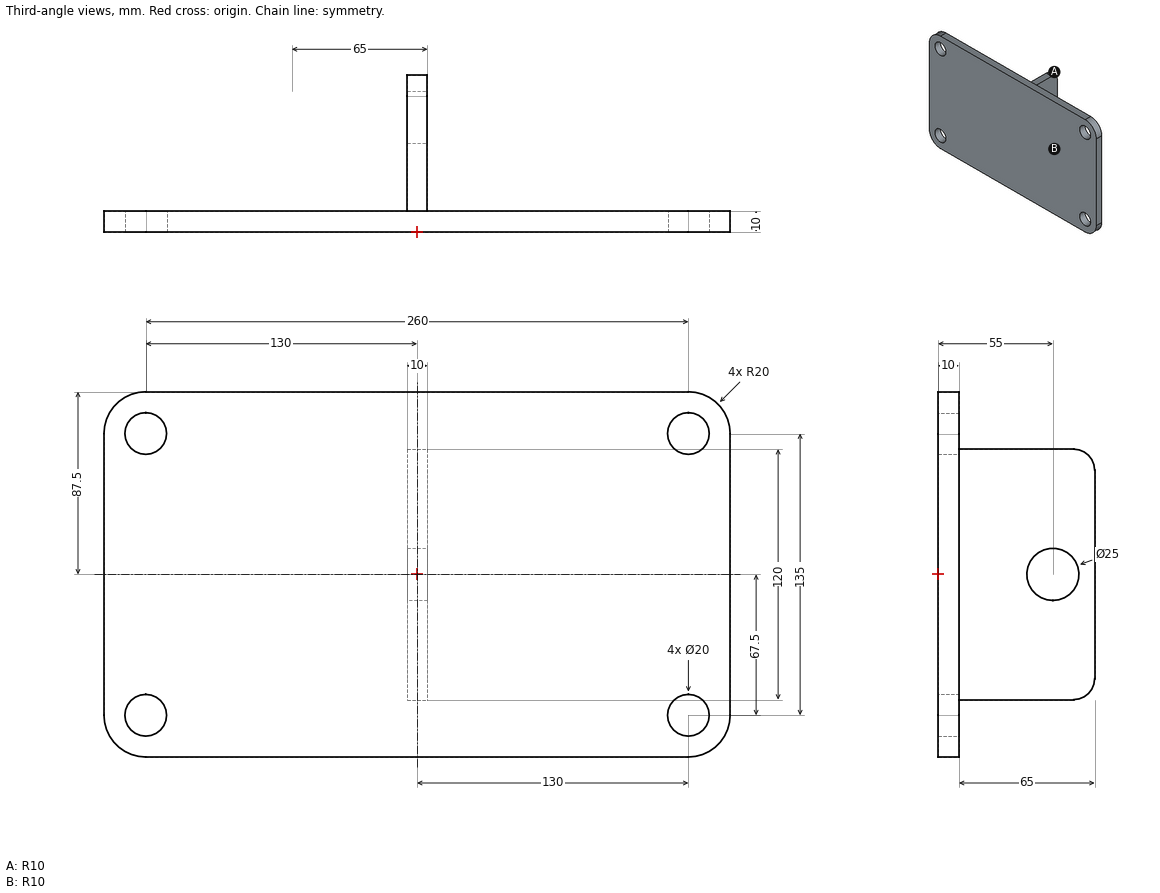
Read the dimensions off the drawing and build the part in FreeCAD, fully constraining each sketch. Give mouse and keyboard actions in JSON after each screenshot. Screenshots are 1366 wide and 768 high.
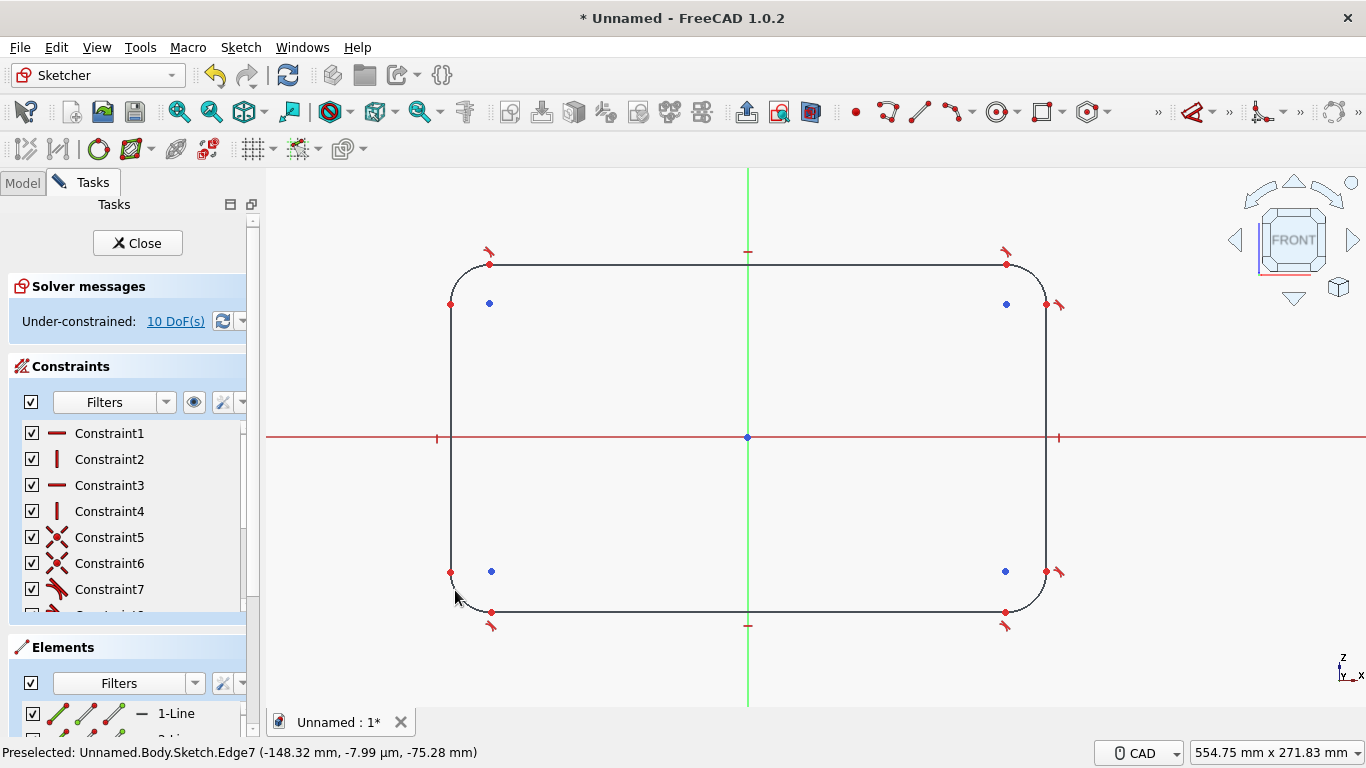
{"action": "left_click", "coordinate": [451, 492]}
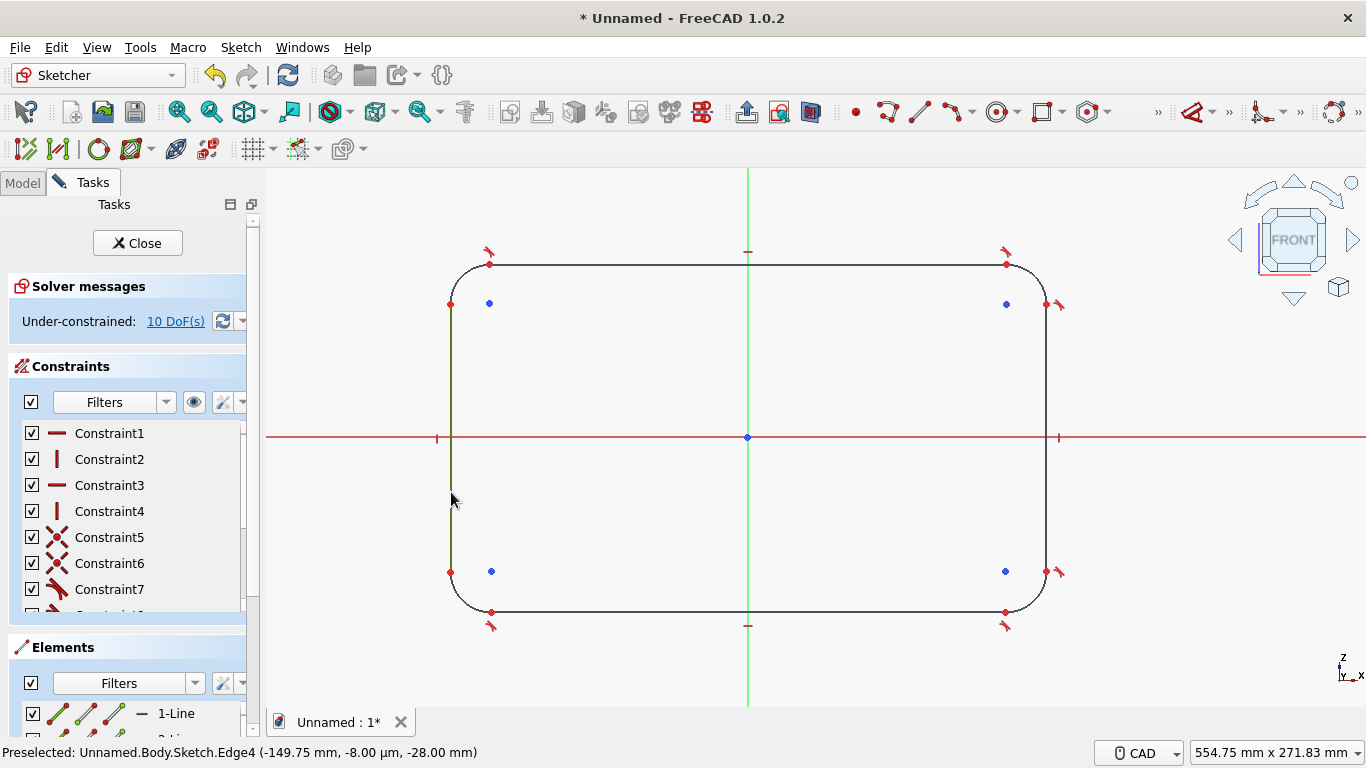
{"action": "left_click", "coordinate": [455, 591]}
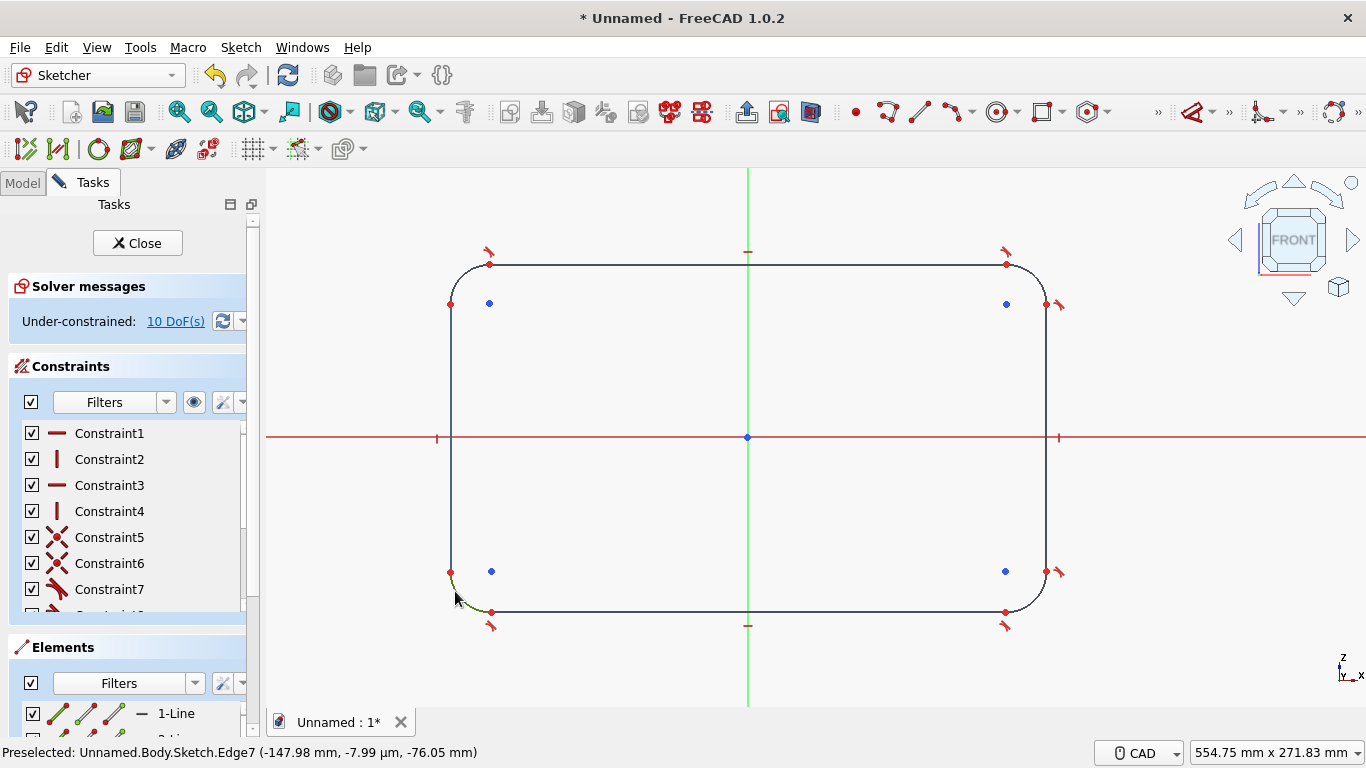
{"action": "key", "text": "t"}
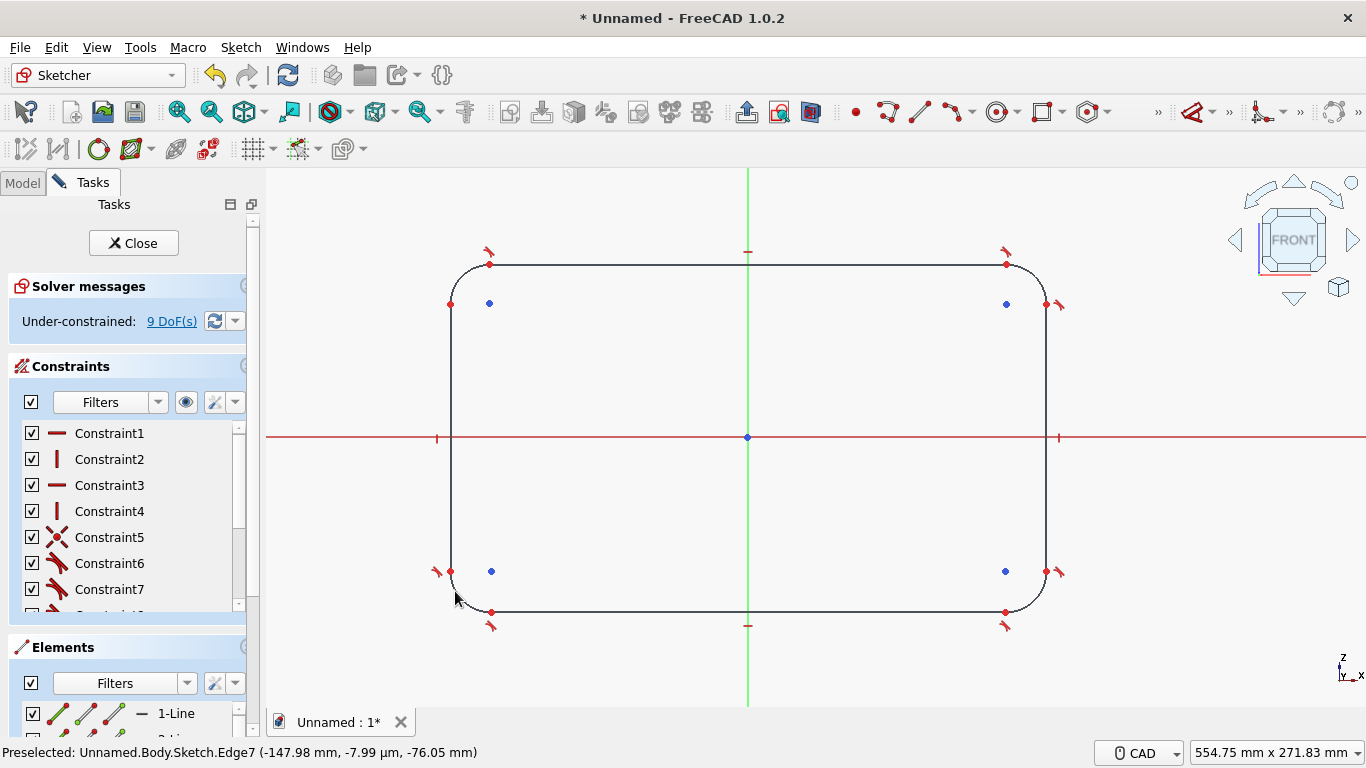
{"action": "left_click", "coordinate": [451, 491]}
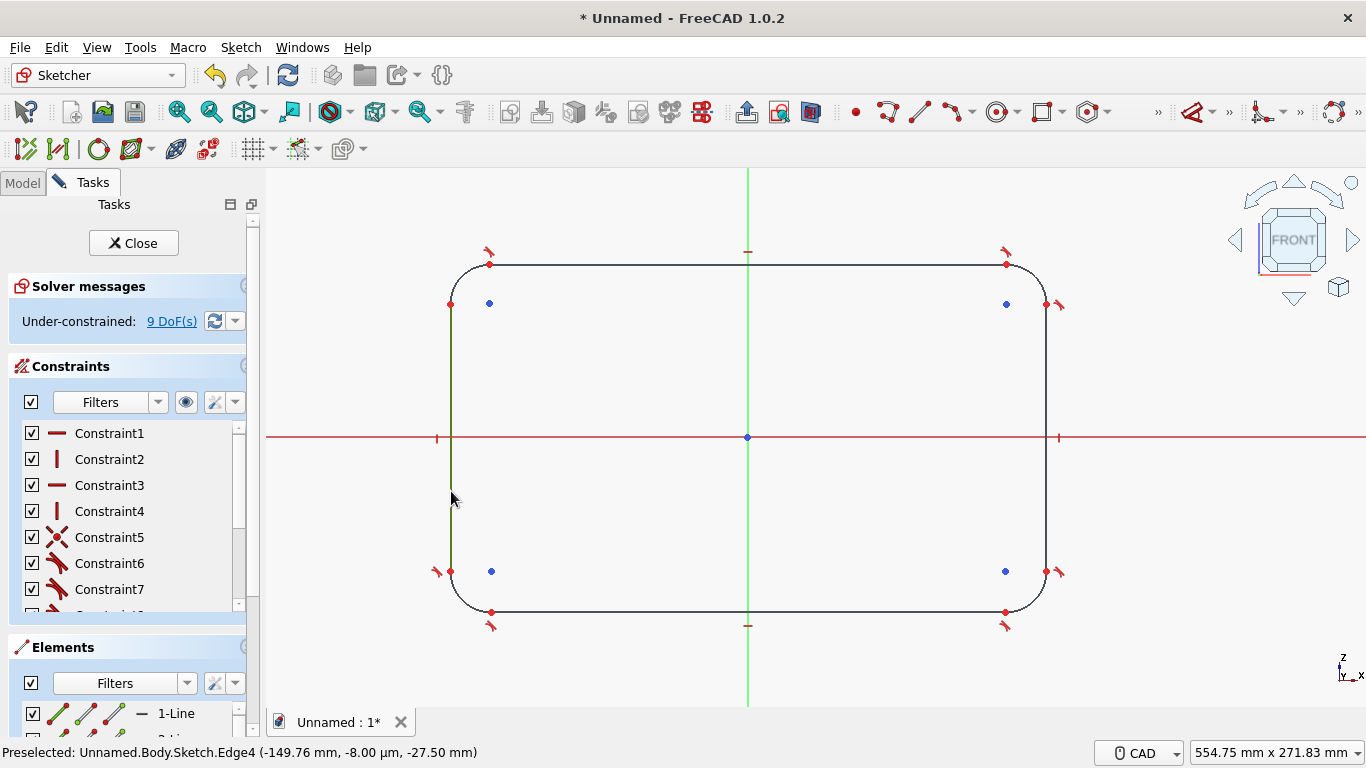
{"action": "left_click", "coordinate": [472, 269]}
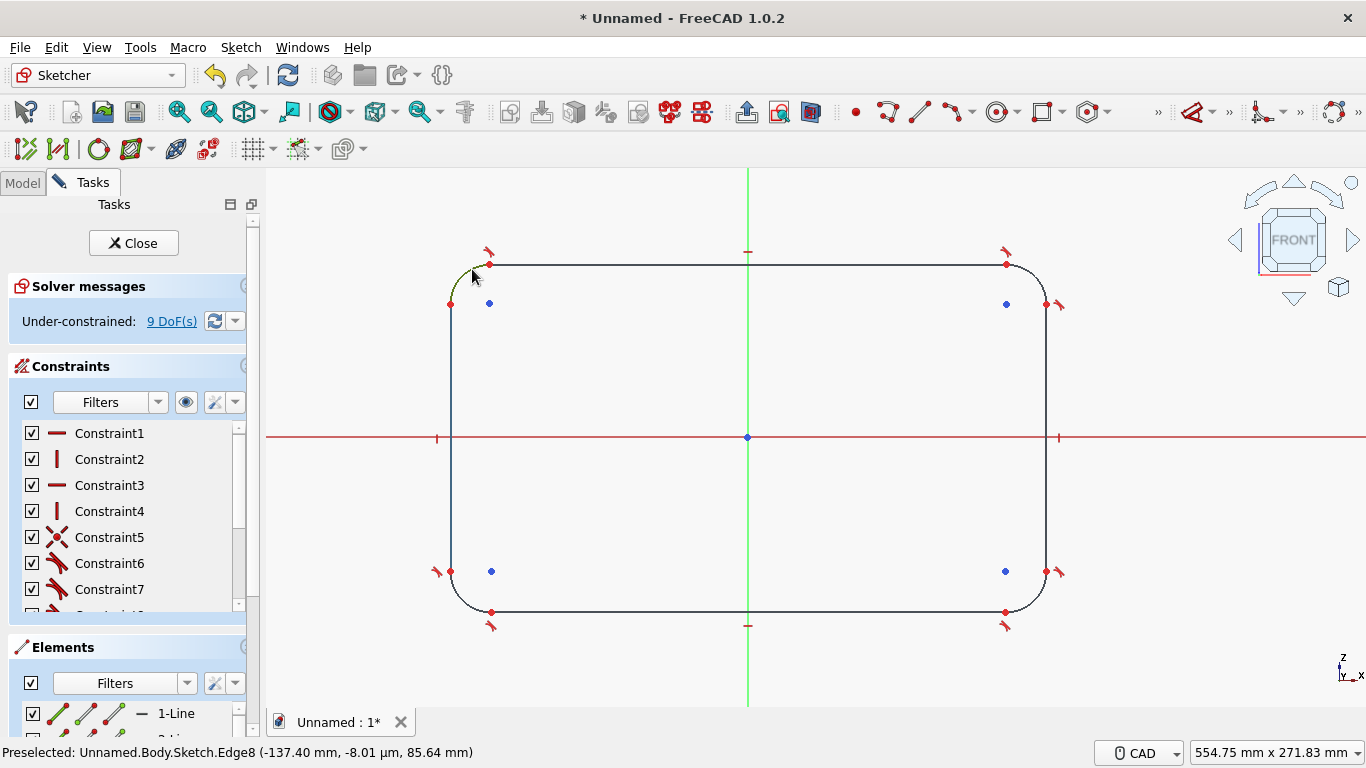
{"action": "key", "text": "t"}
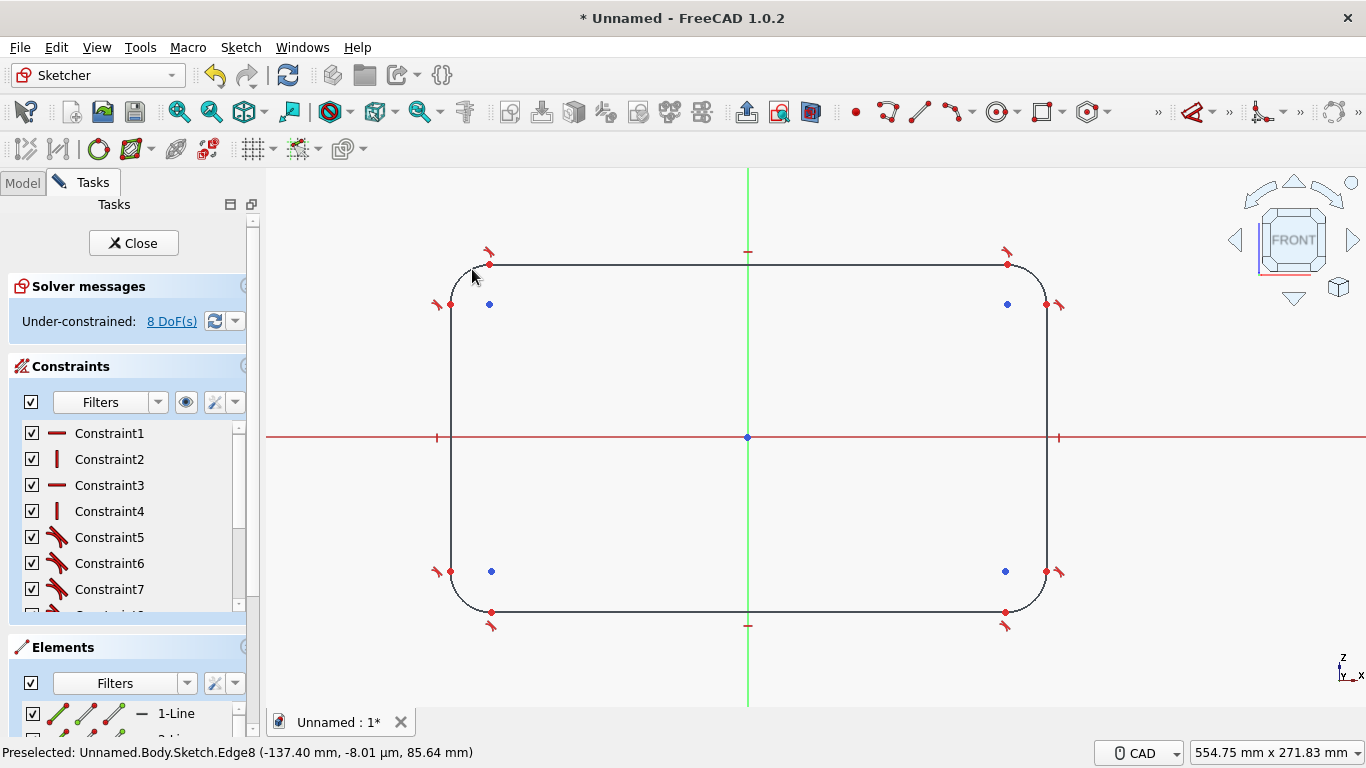
{"action": "left_click", "coordinate": [1042, 286]}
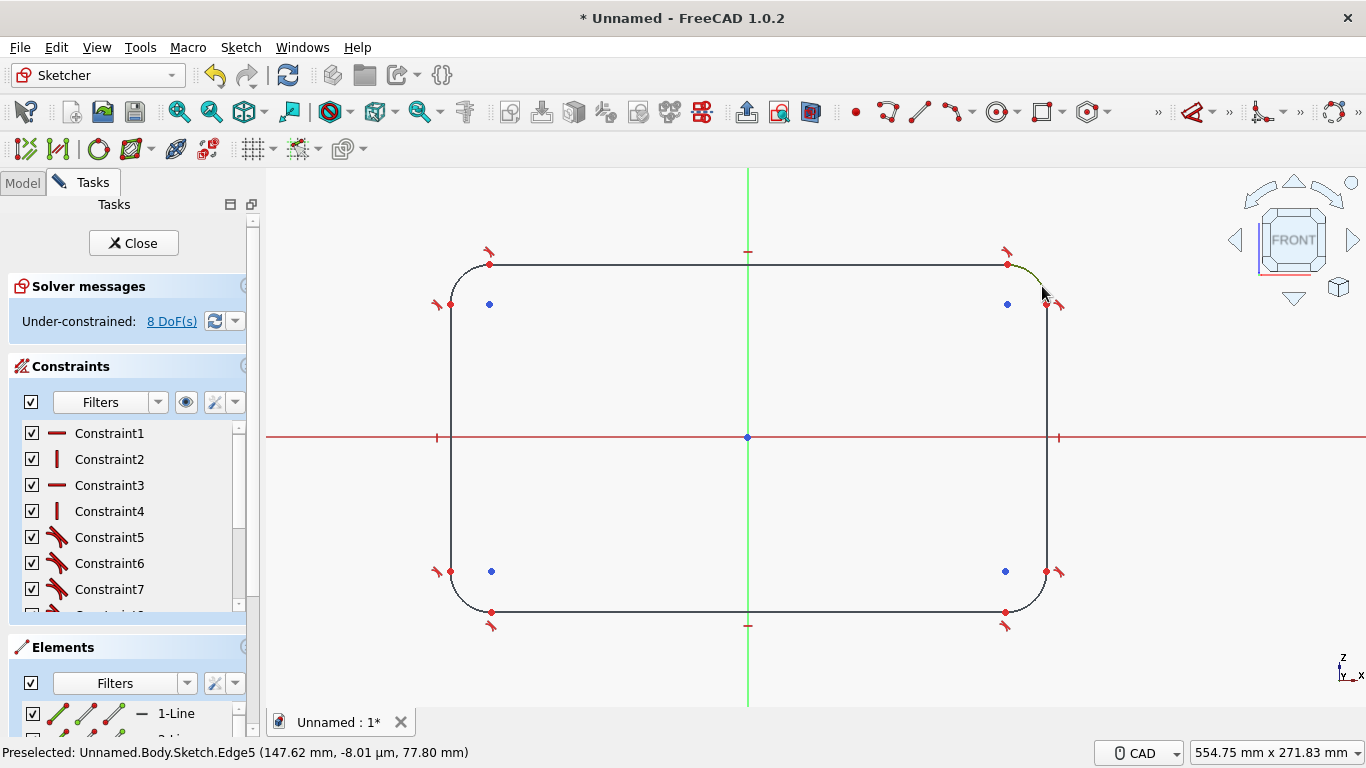
{"action": "left_click", "coordinate": [1024, 608]}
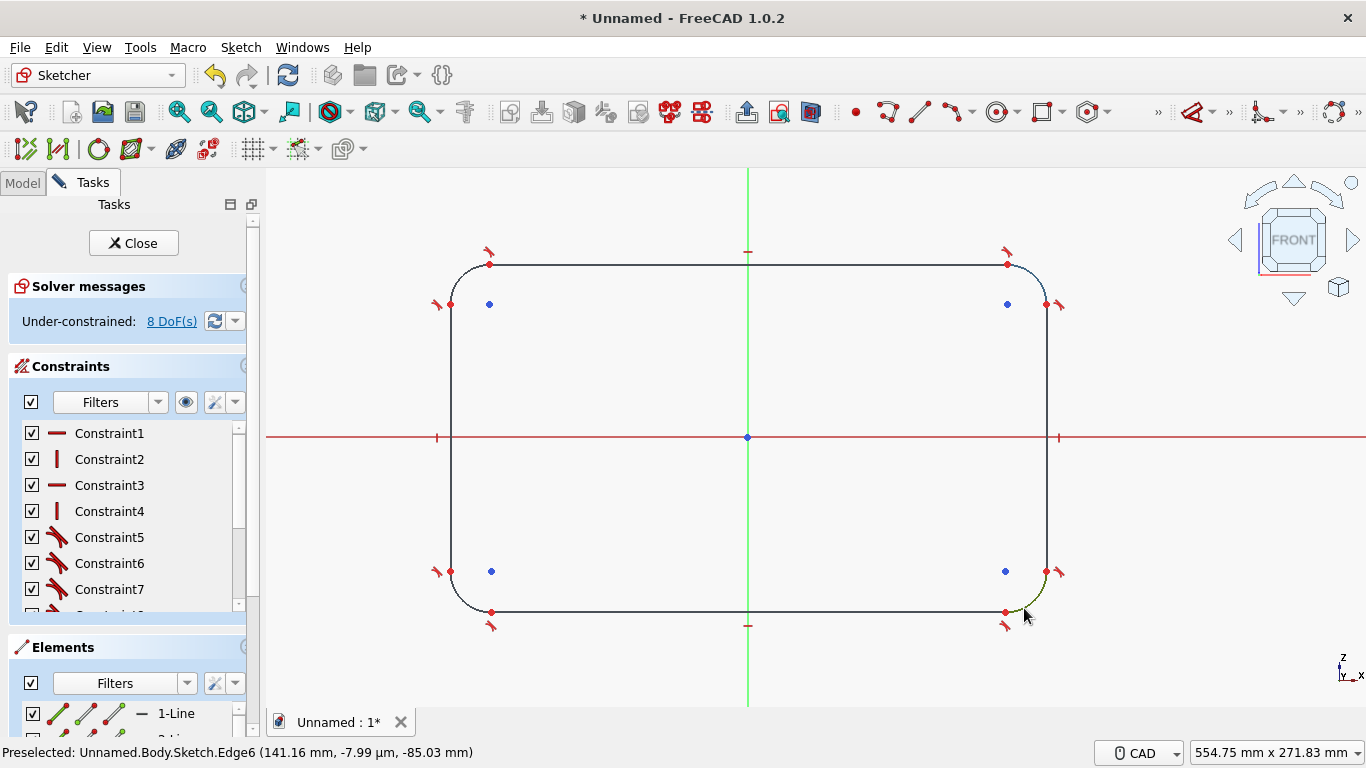
{"action": "left_click", "coordinate": [455, 590]}